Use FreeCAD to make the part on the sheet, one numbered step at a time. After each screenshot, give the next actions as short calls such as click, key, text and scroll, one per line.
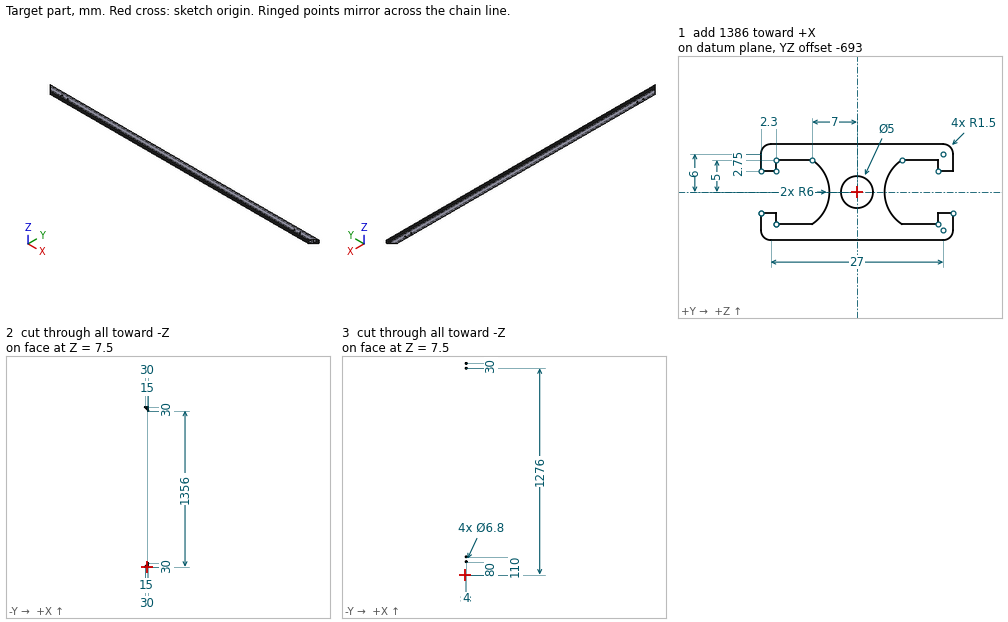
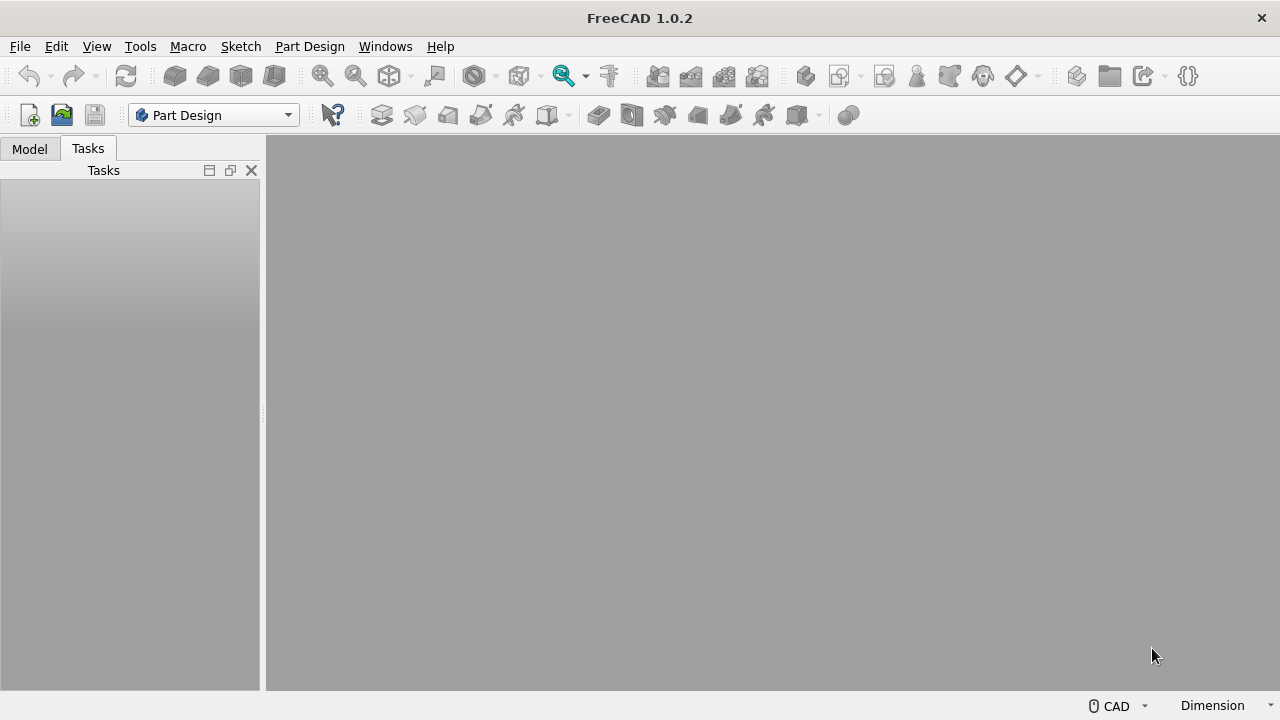
key(ctrl+n)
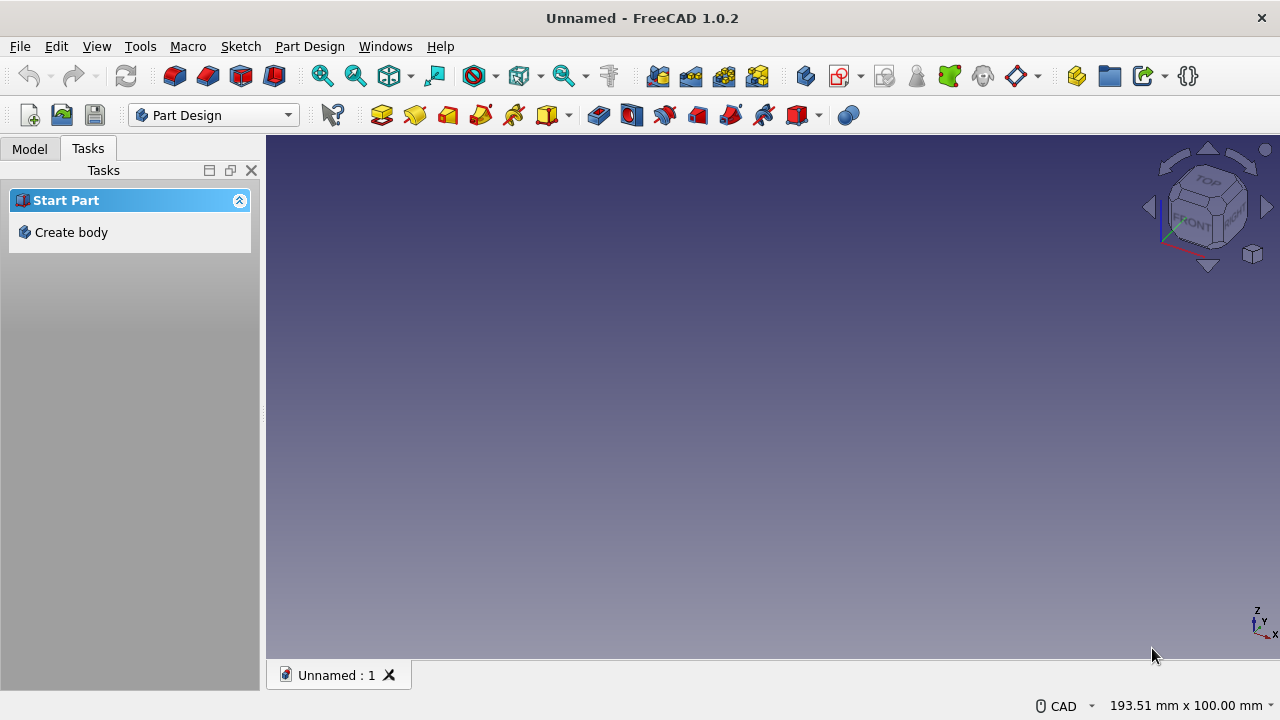
click(806, 76)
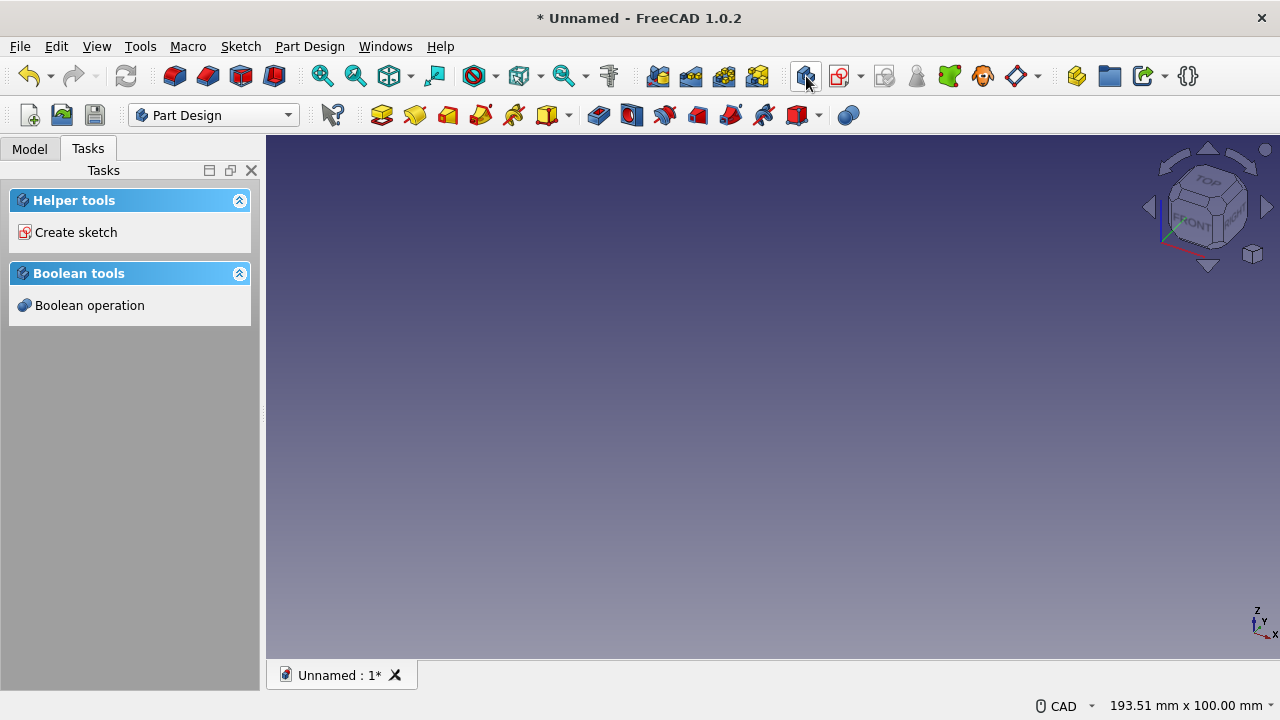
click(30, 148)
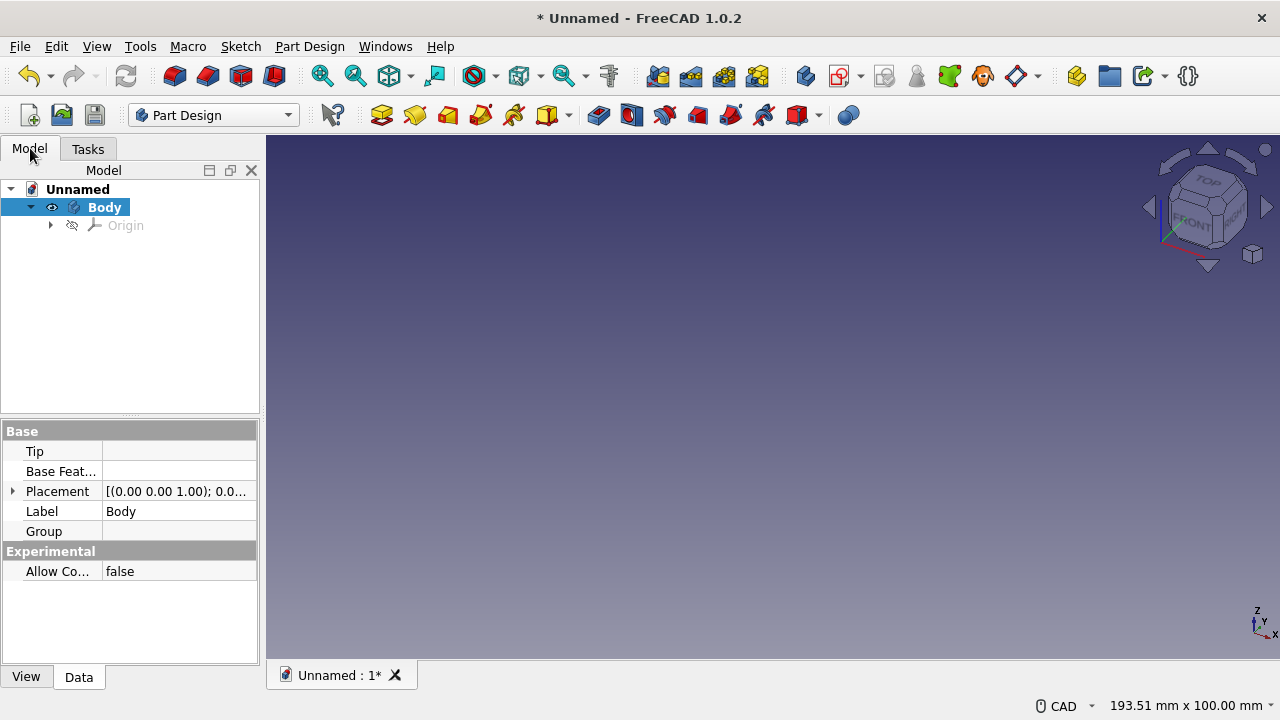
click(51, 225)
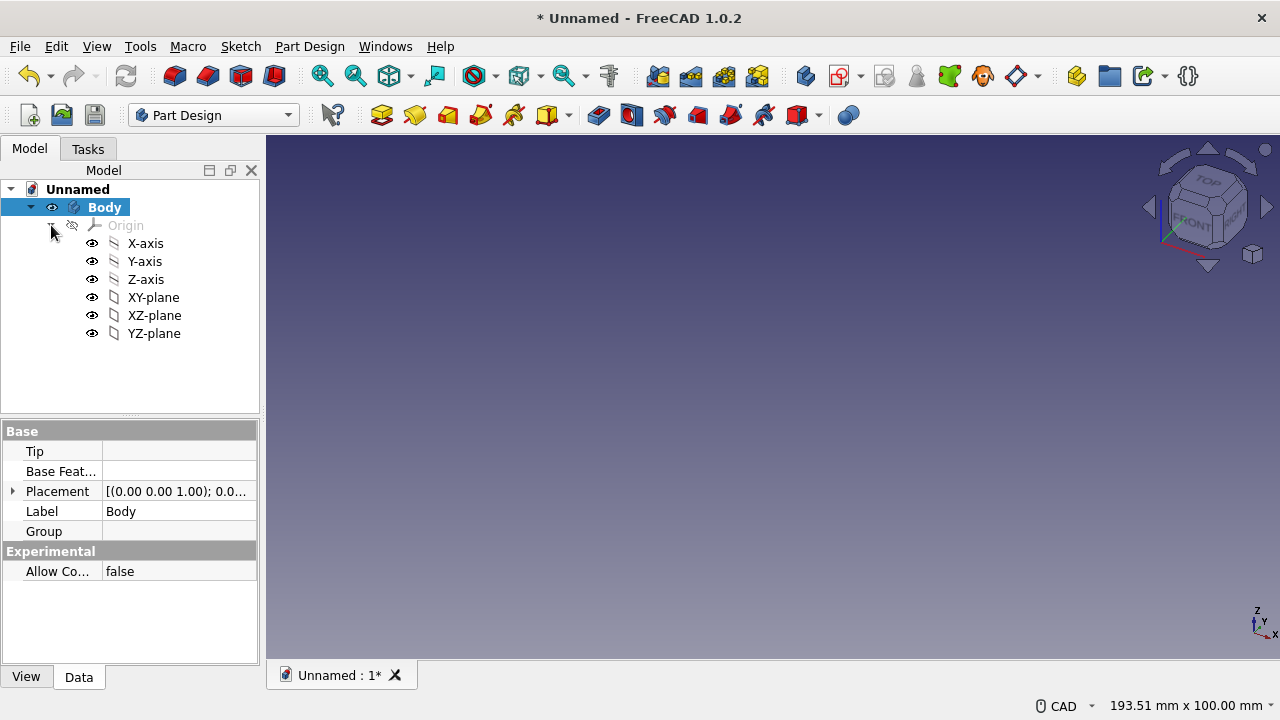
click(137, 333)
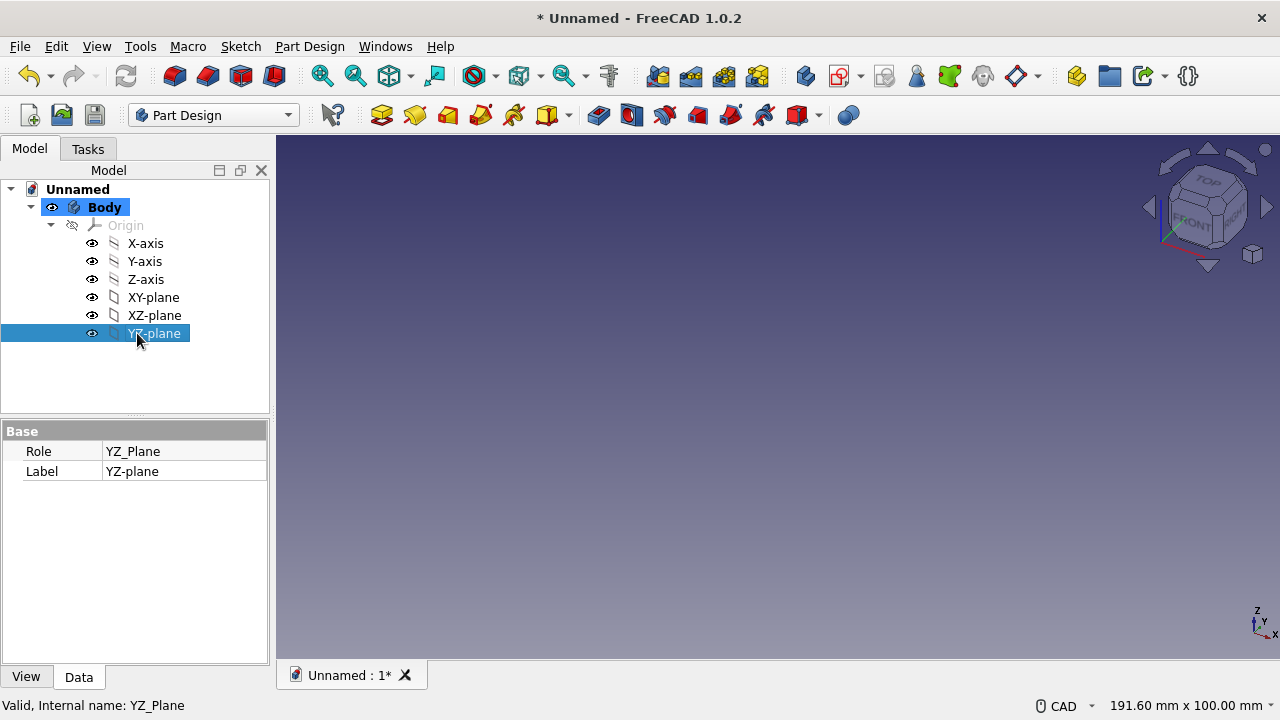
click(1016, 76)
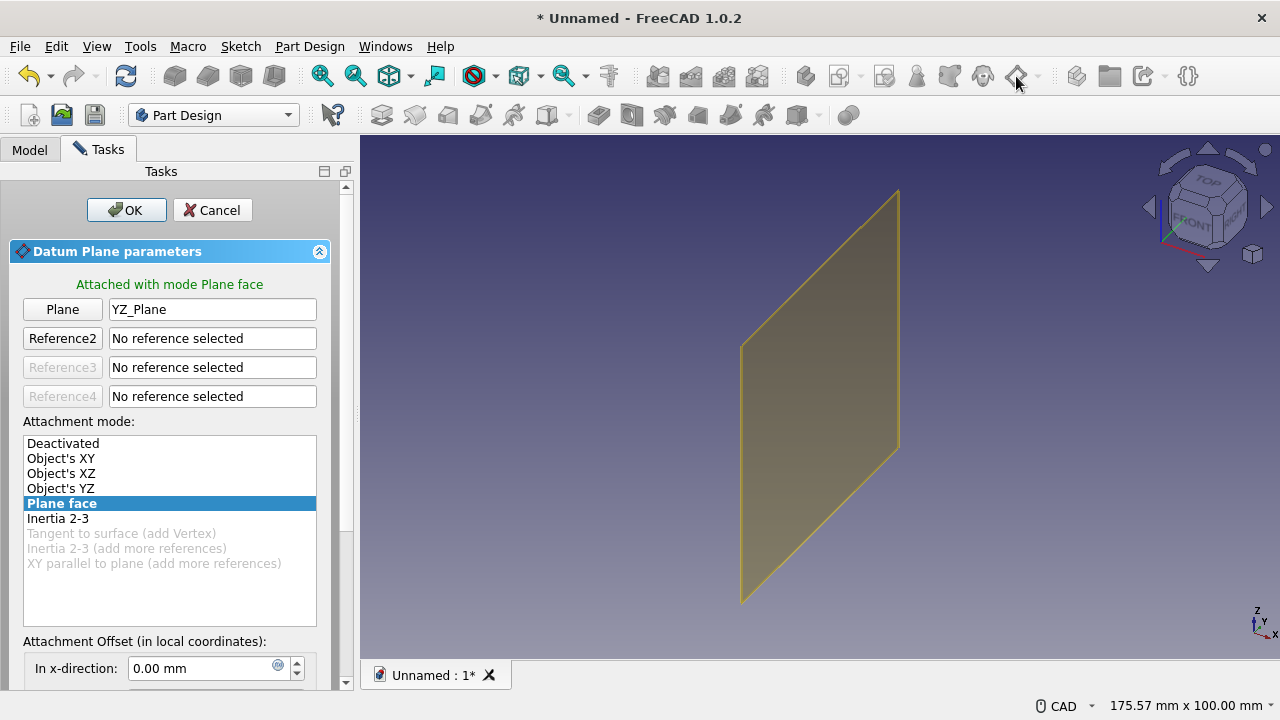
scroll(346, 436, down, 2)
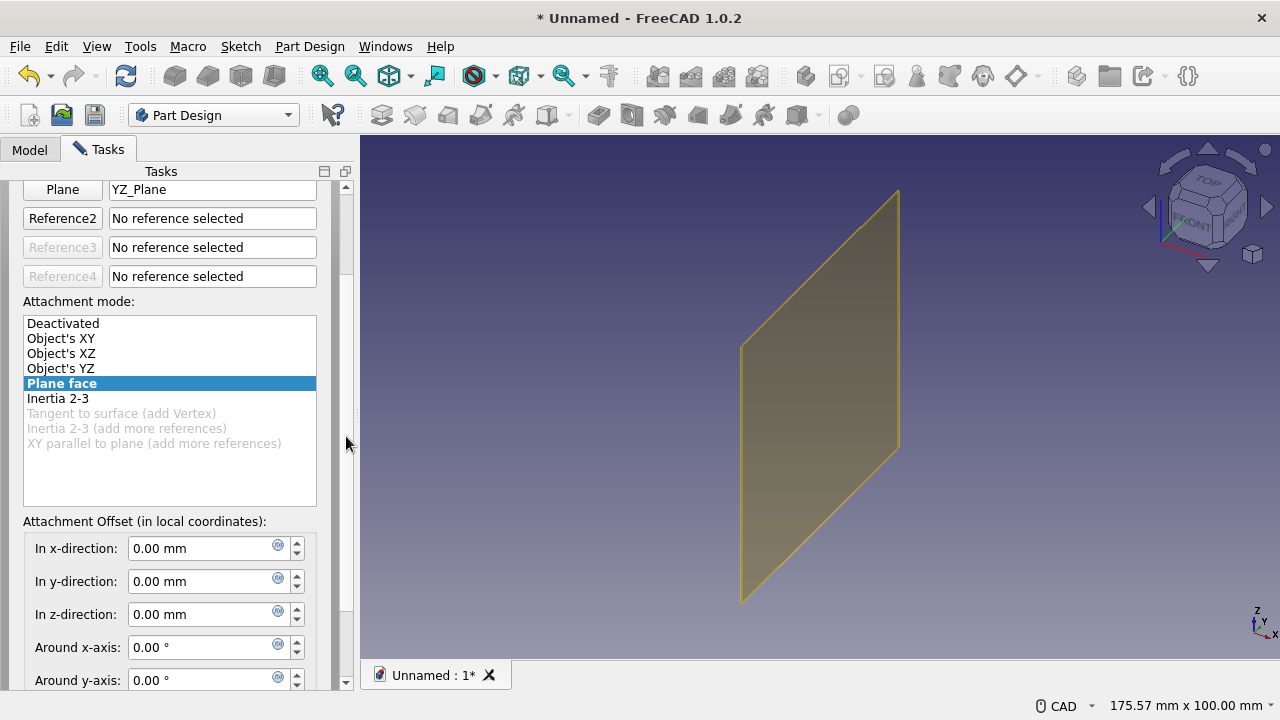
triple_click(210, 614)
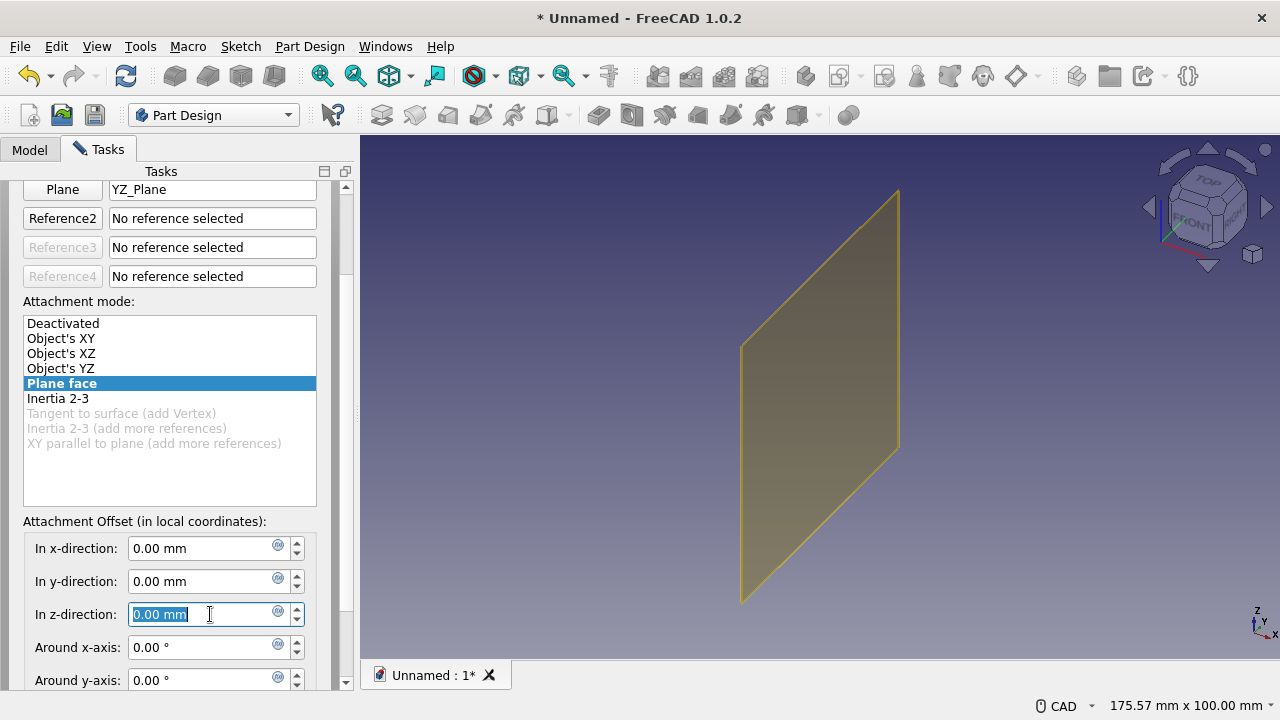
text(-693)
key(Tab)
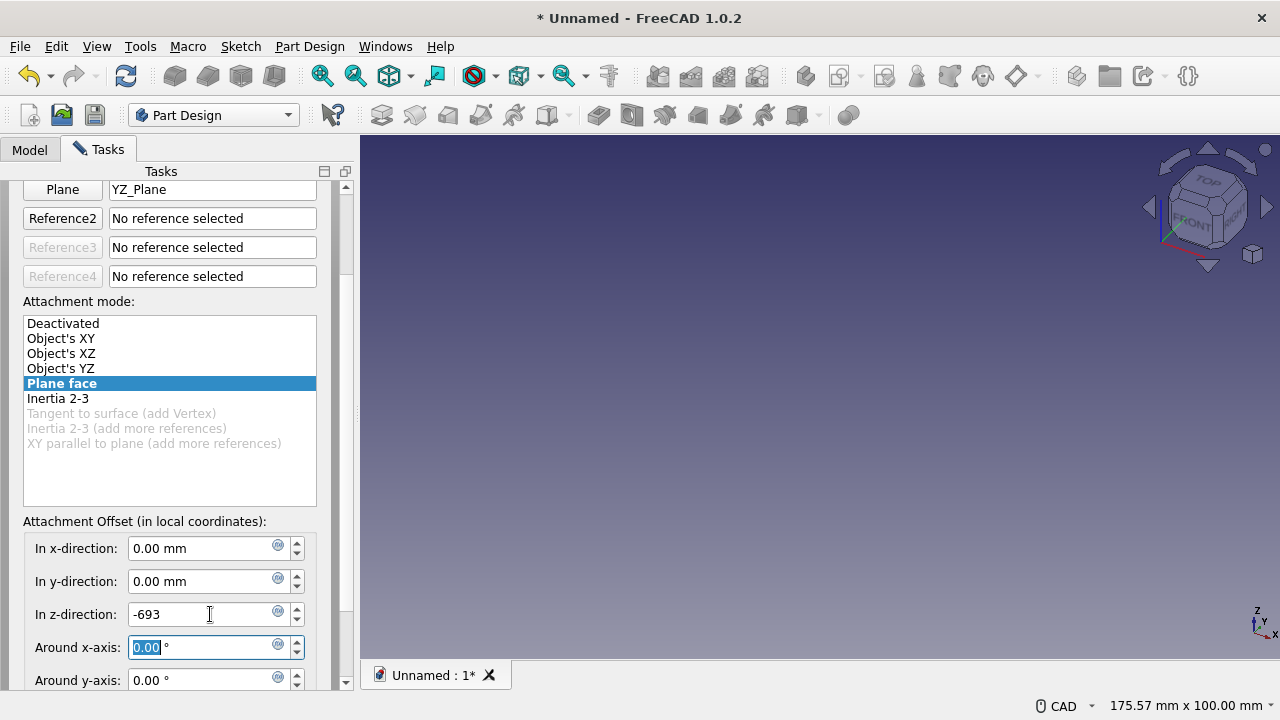
scroll(346, 436, up, 3)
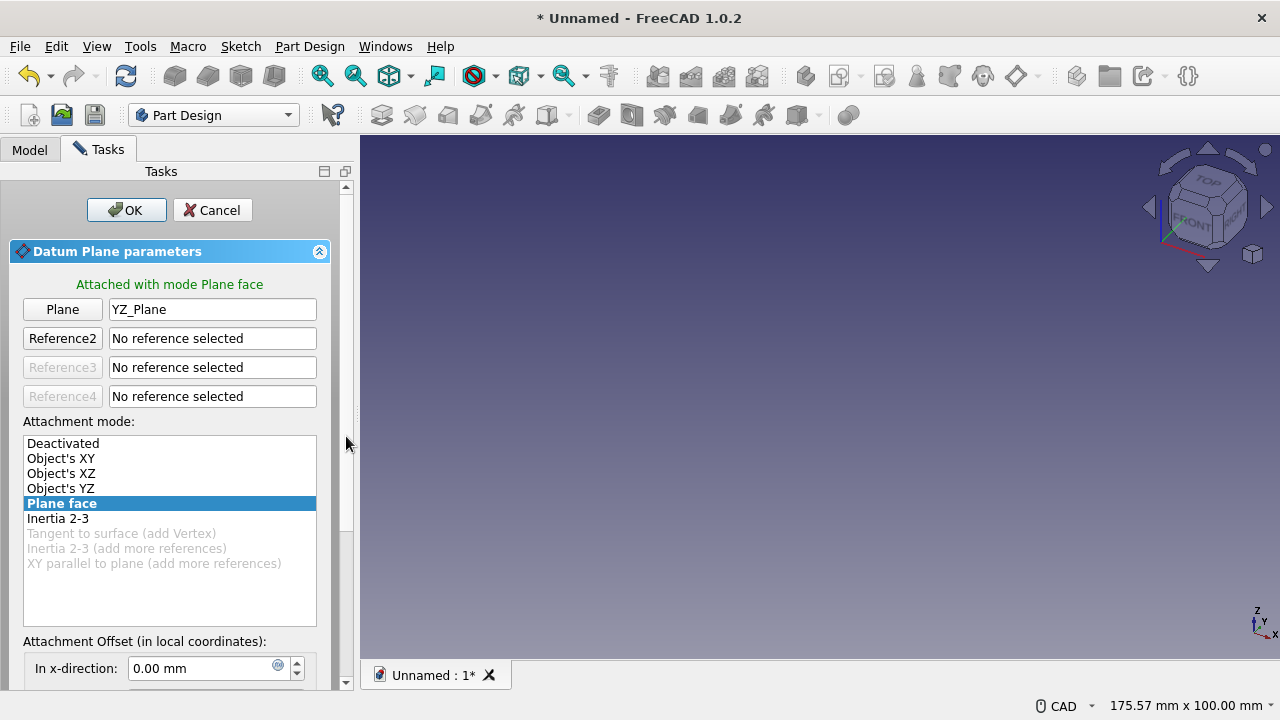
click(127, 210)